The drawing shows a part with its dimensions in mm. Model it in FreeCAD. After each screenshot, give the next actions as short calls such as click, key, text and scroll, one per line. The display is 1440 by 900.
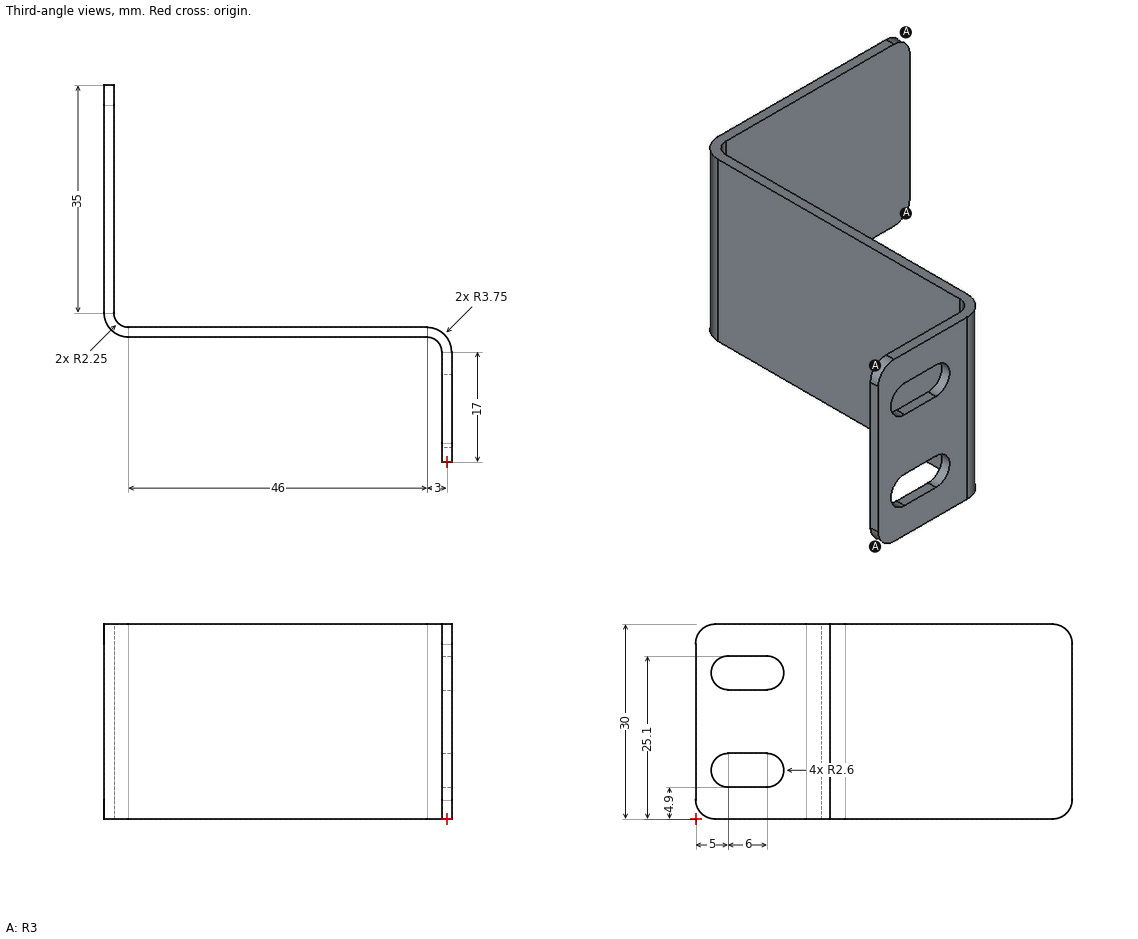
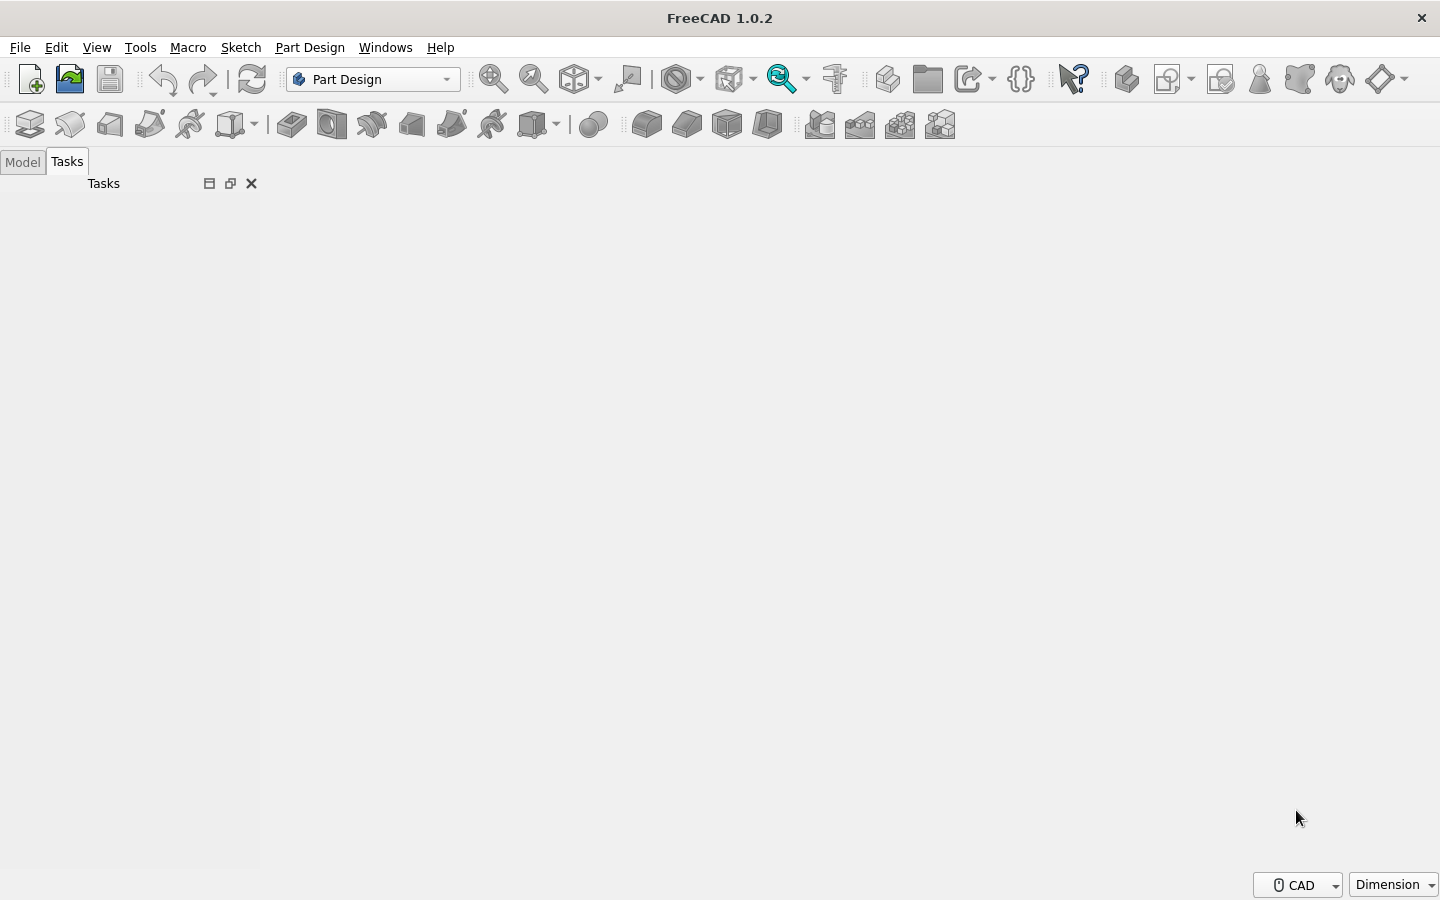
key(ctrl+n)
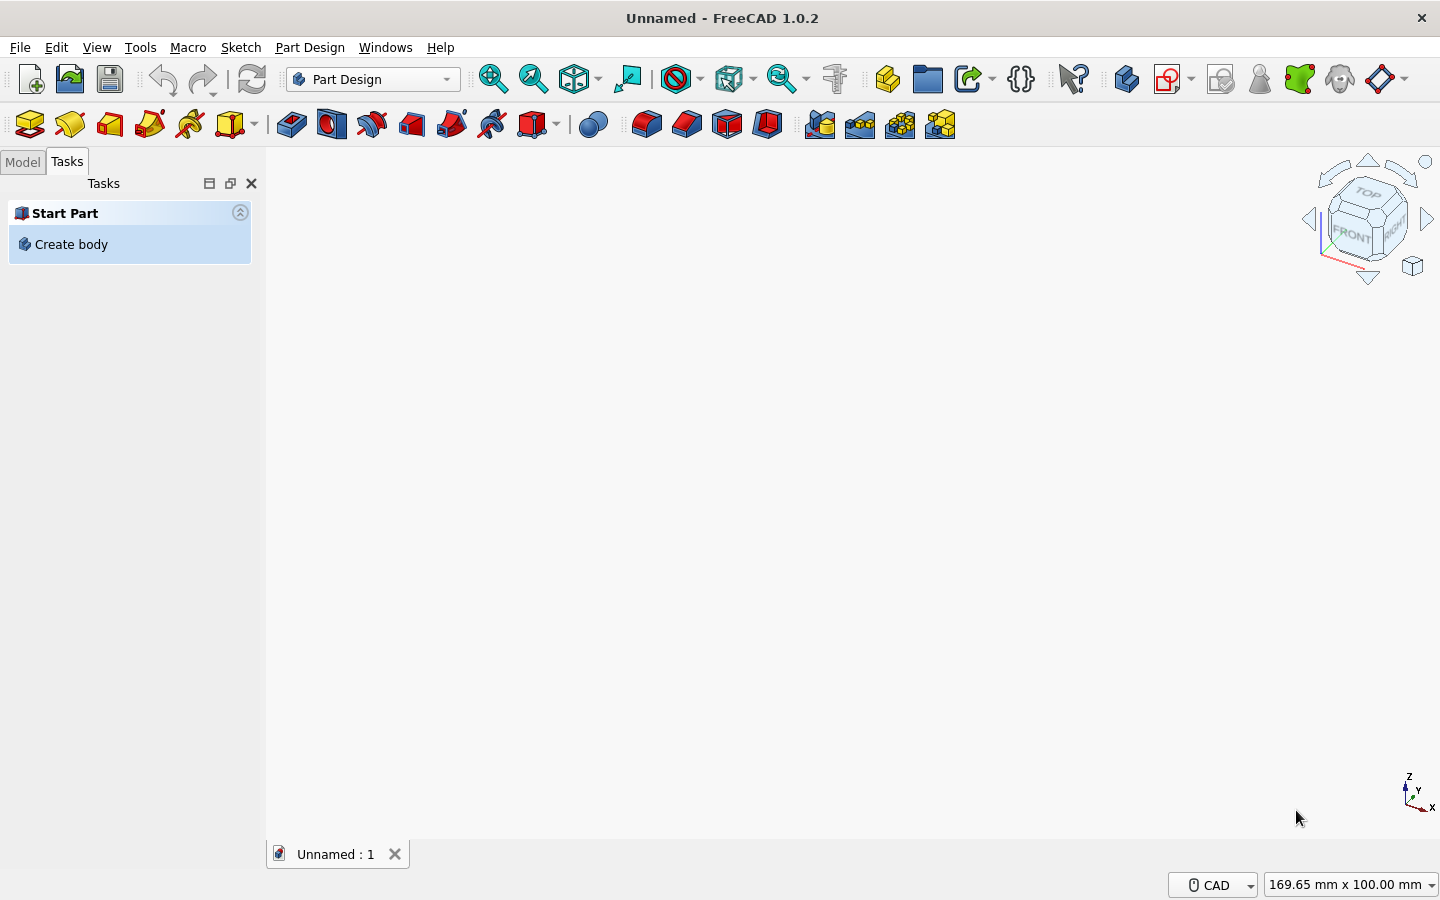
click(1168, 80)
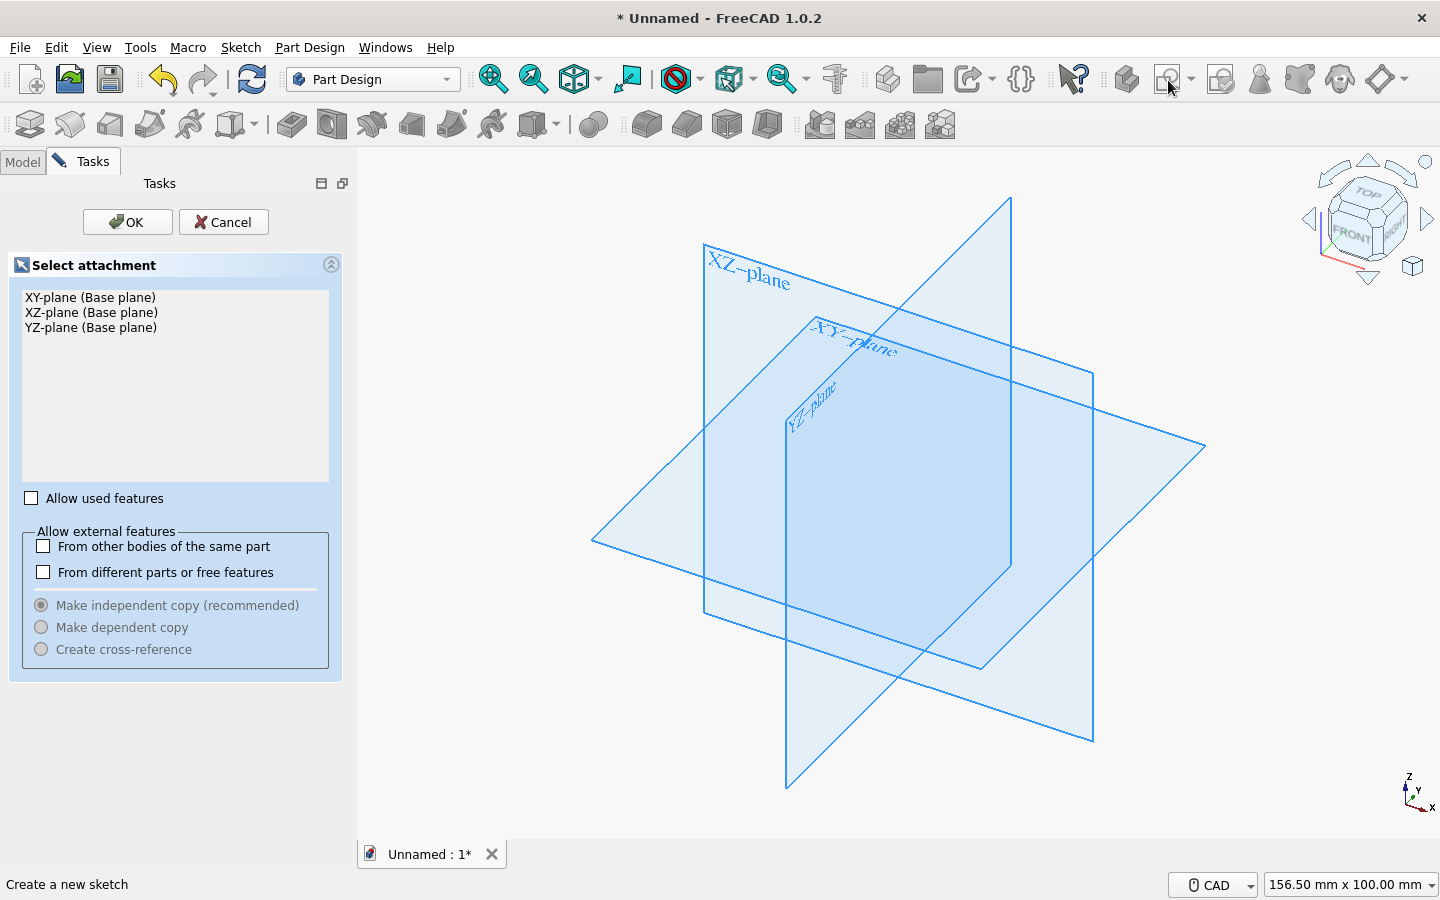
click(82, 298)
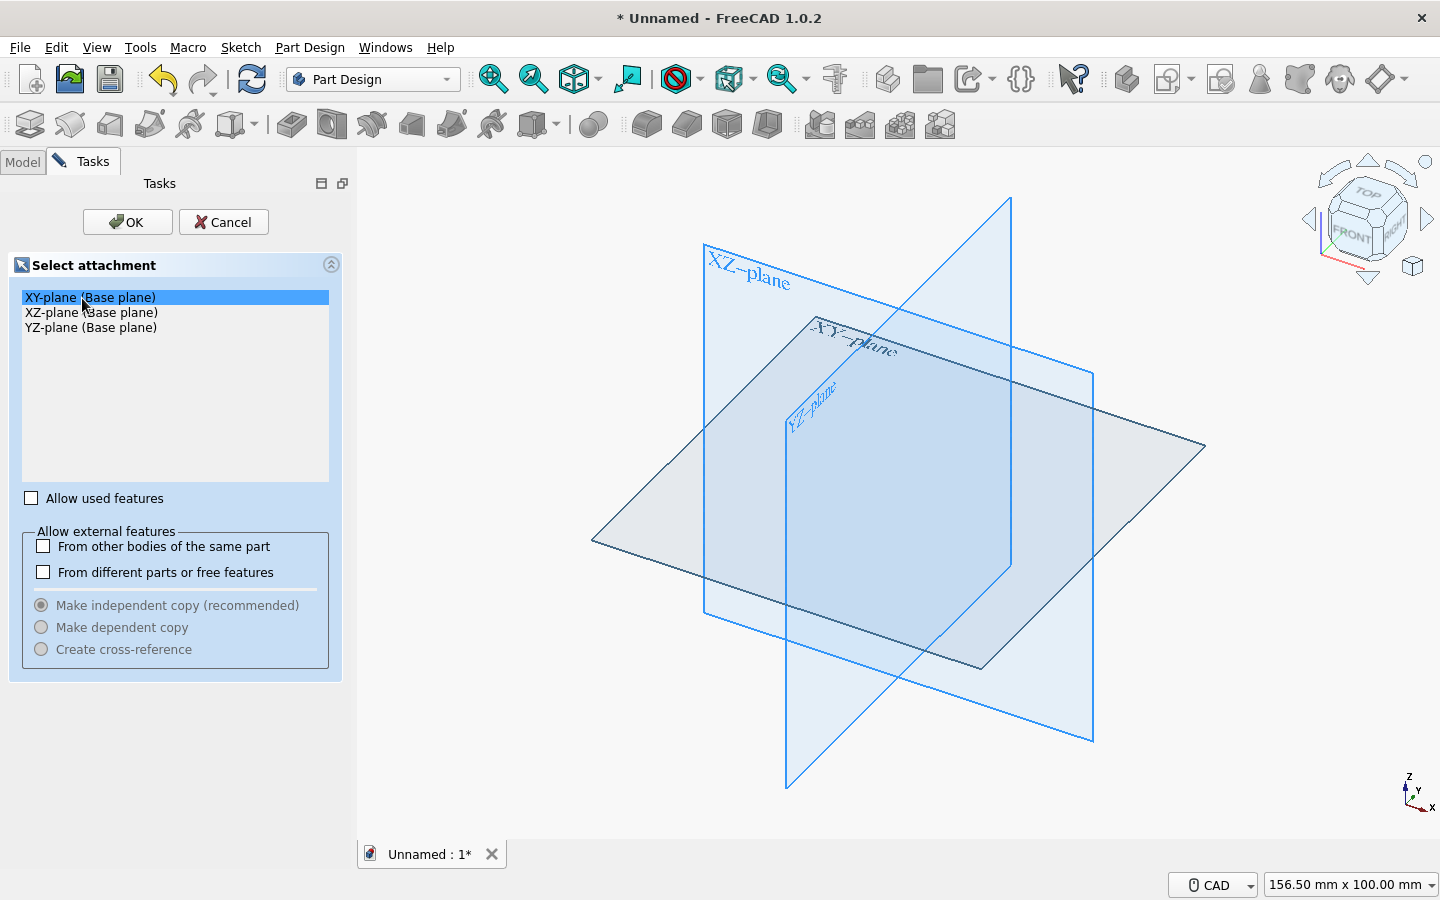
click(128, 222)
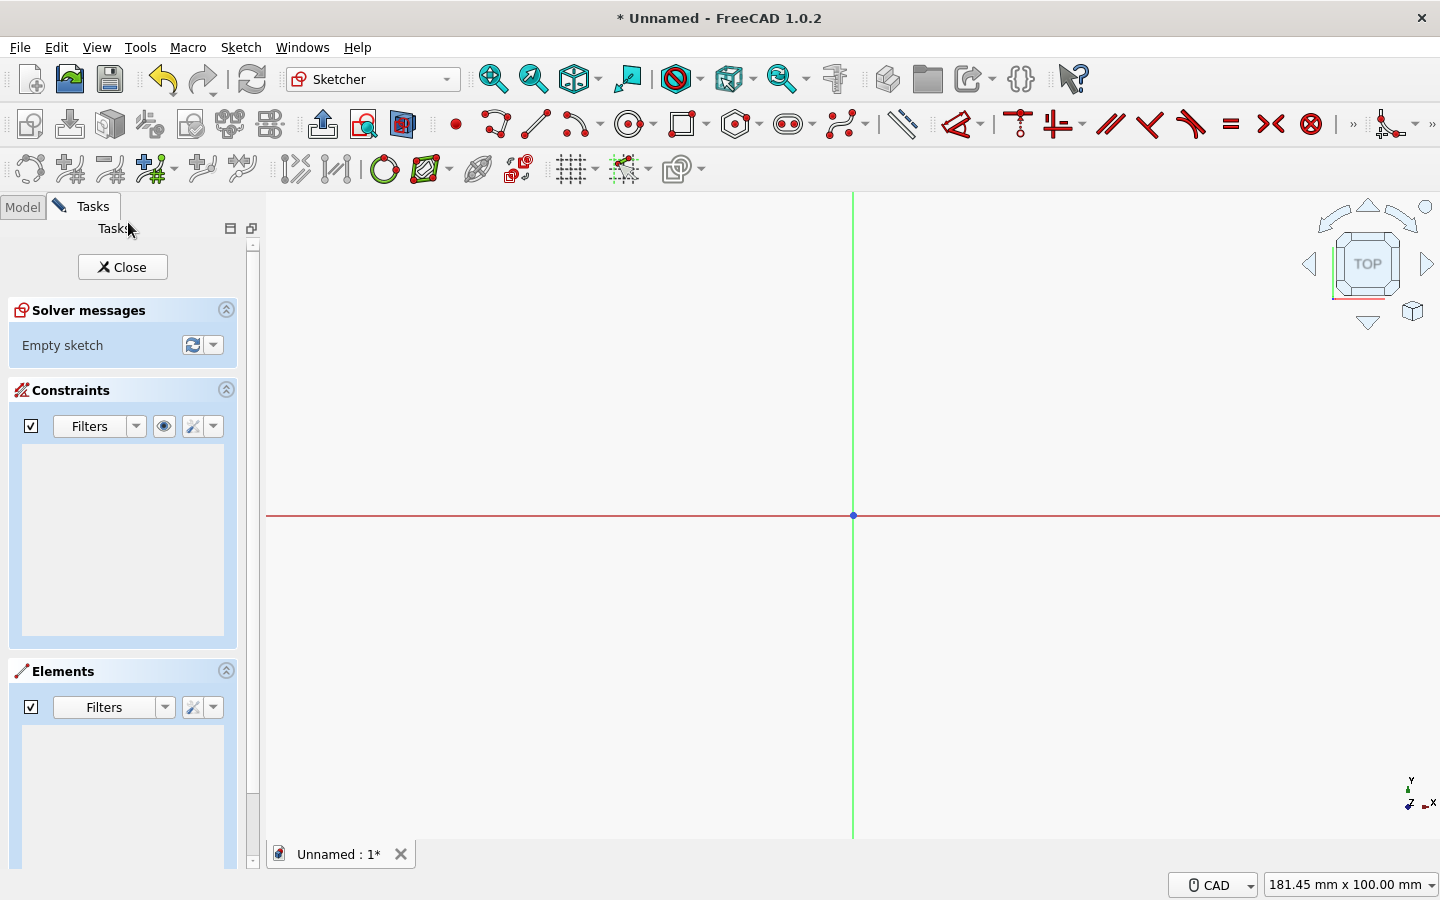
scroll(1235, 811, down, 1)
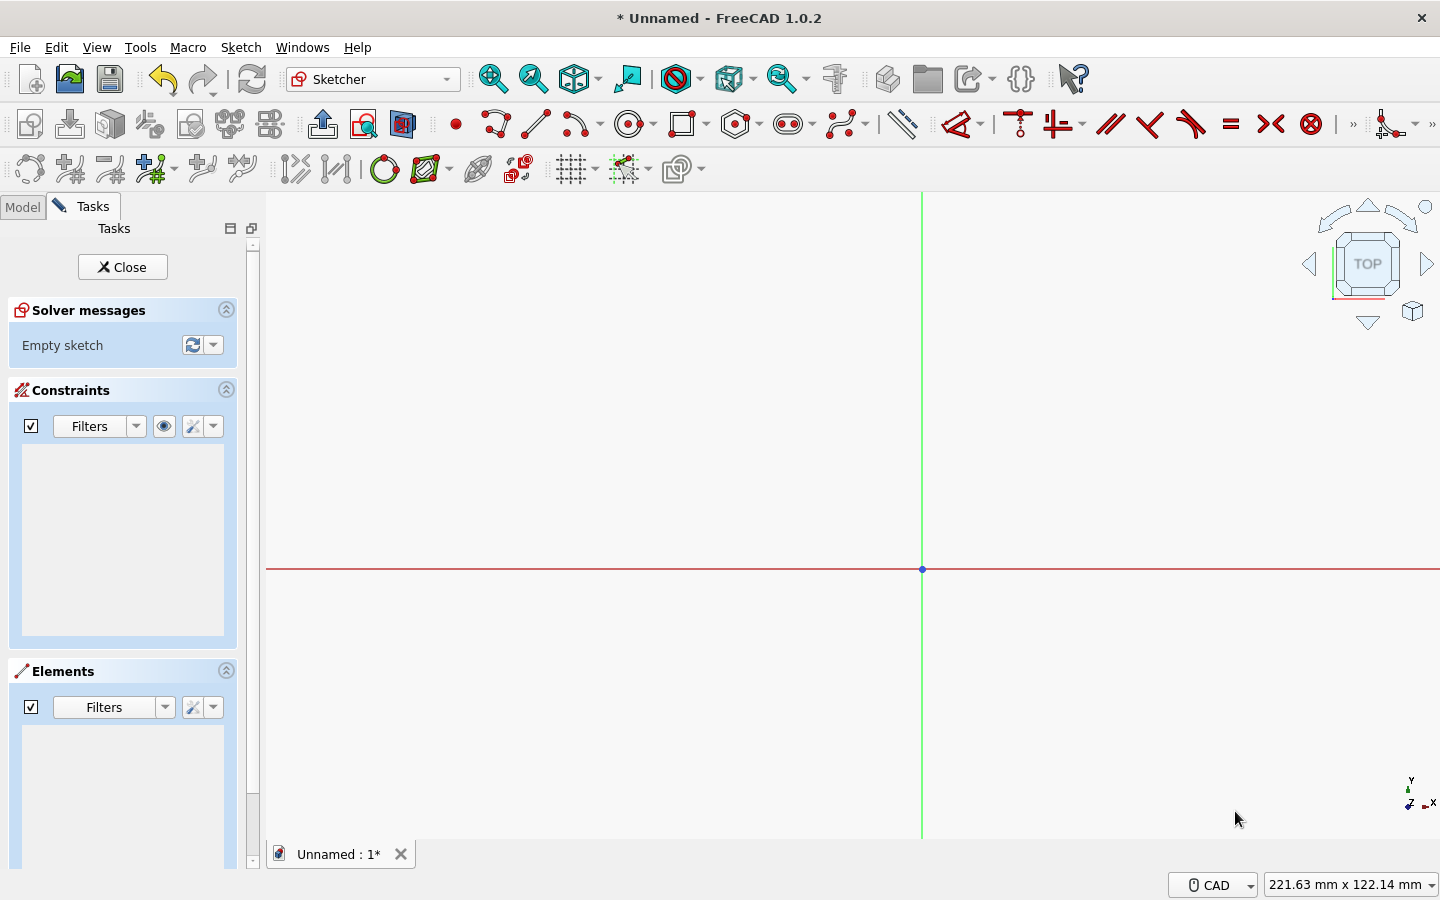
scroll(785, 220, up, 2)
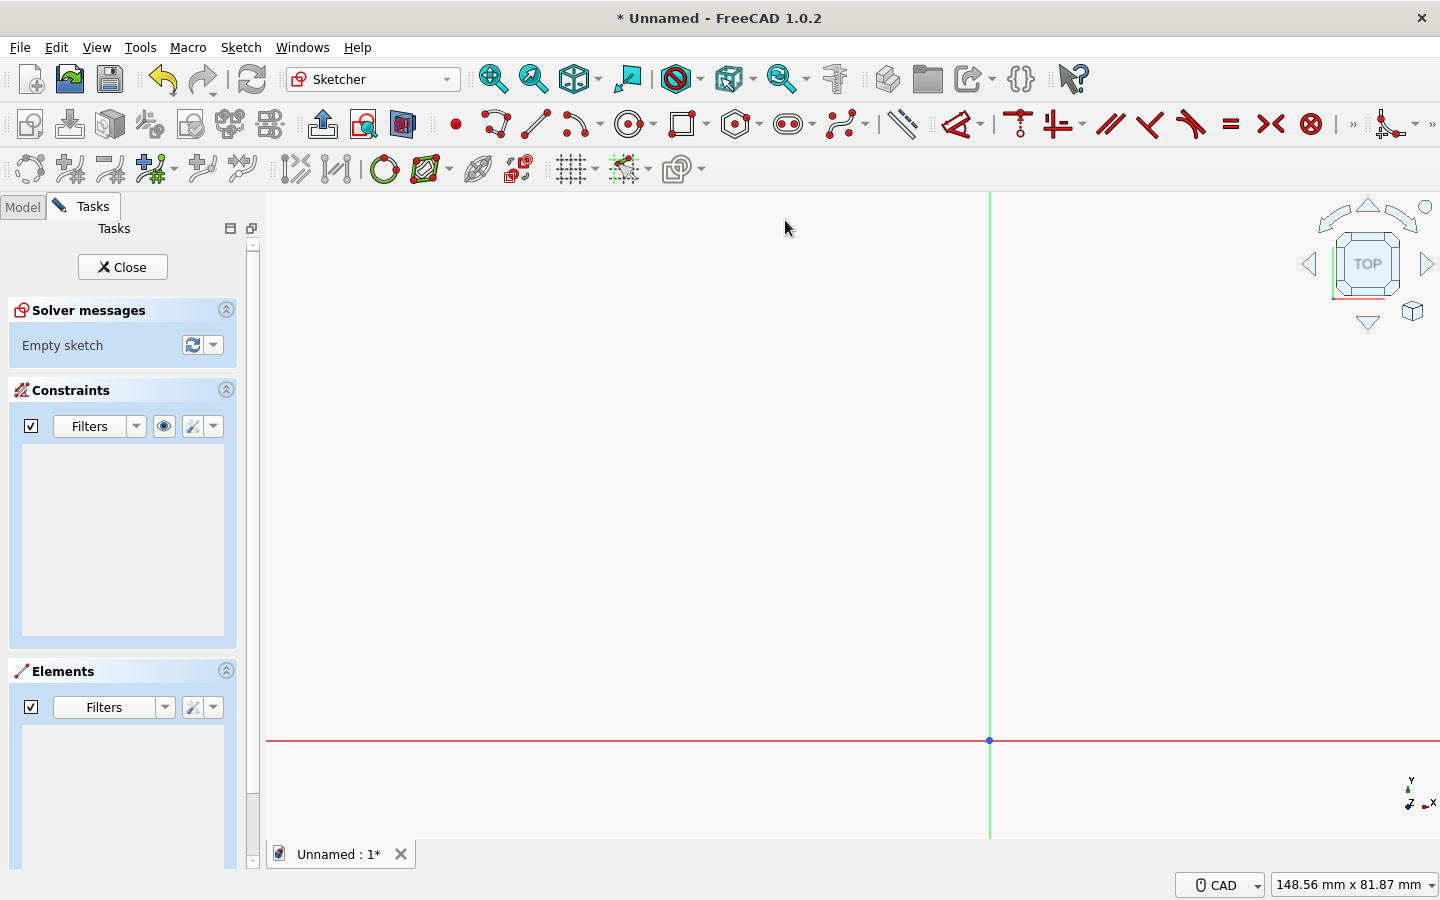
key(g)
key(l)